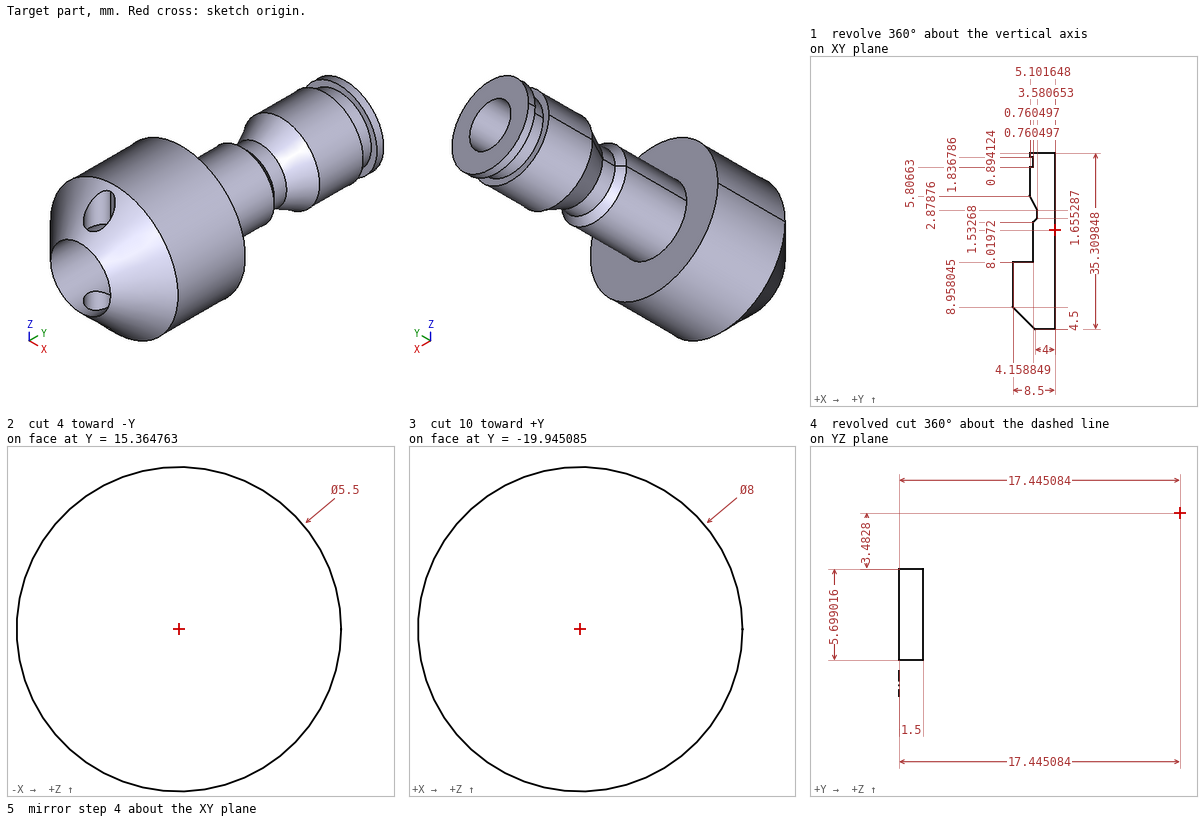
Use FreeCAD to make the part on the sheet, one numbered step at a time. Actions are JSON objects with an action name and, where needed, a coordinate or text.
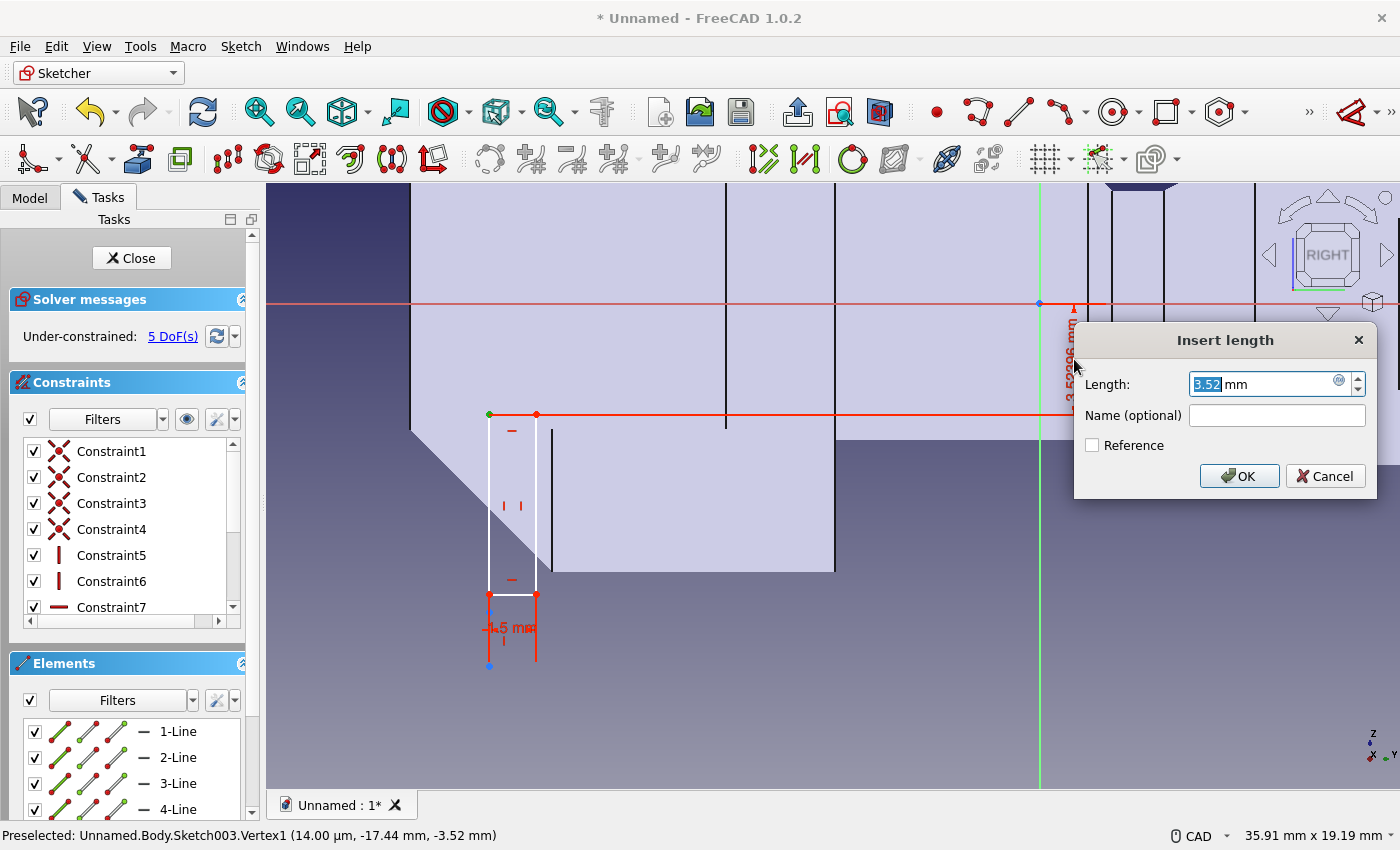
{"action": "type", "text": "3.4828"}
{"action": "key", "text": "Return"}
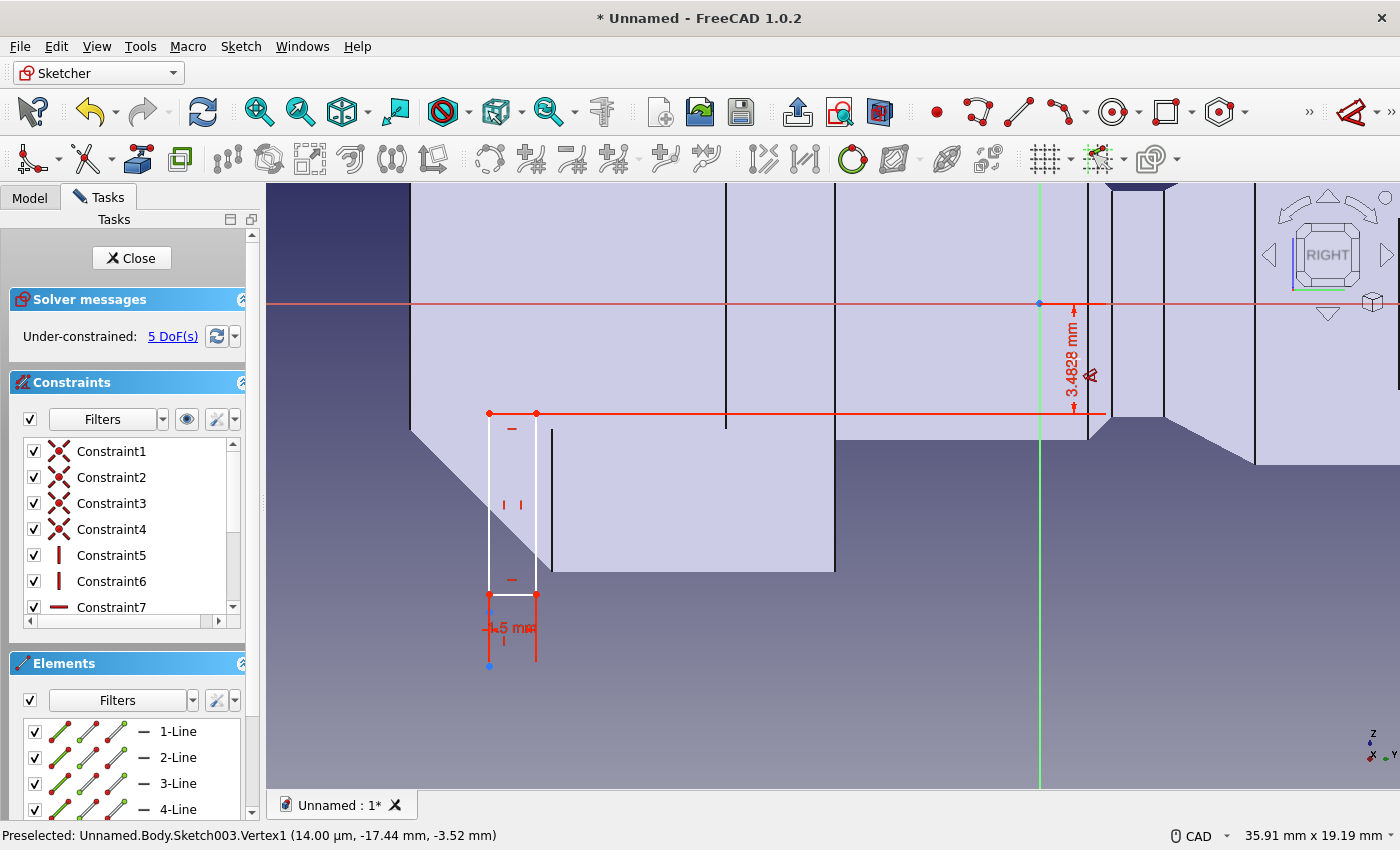
{"action": "left_click", "coordinate": [489, 468]}
{"action": "left_click", "coordinate": [455, 504]}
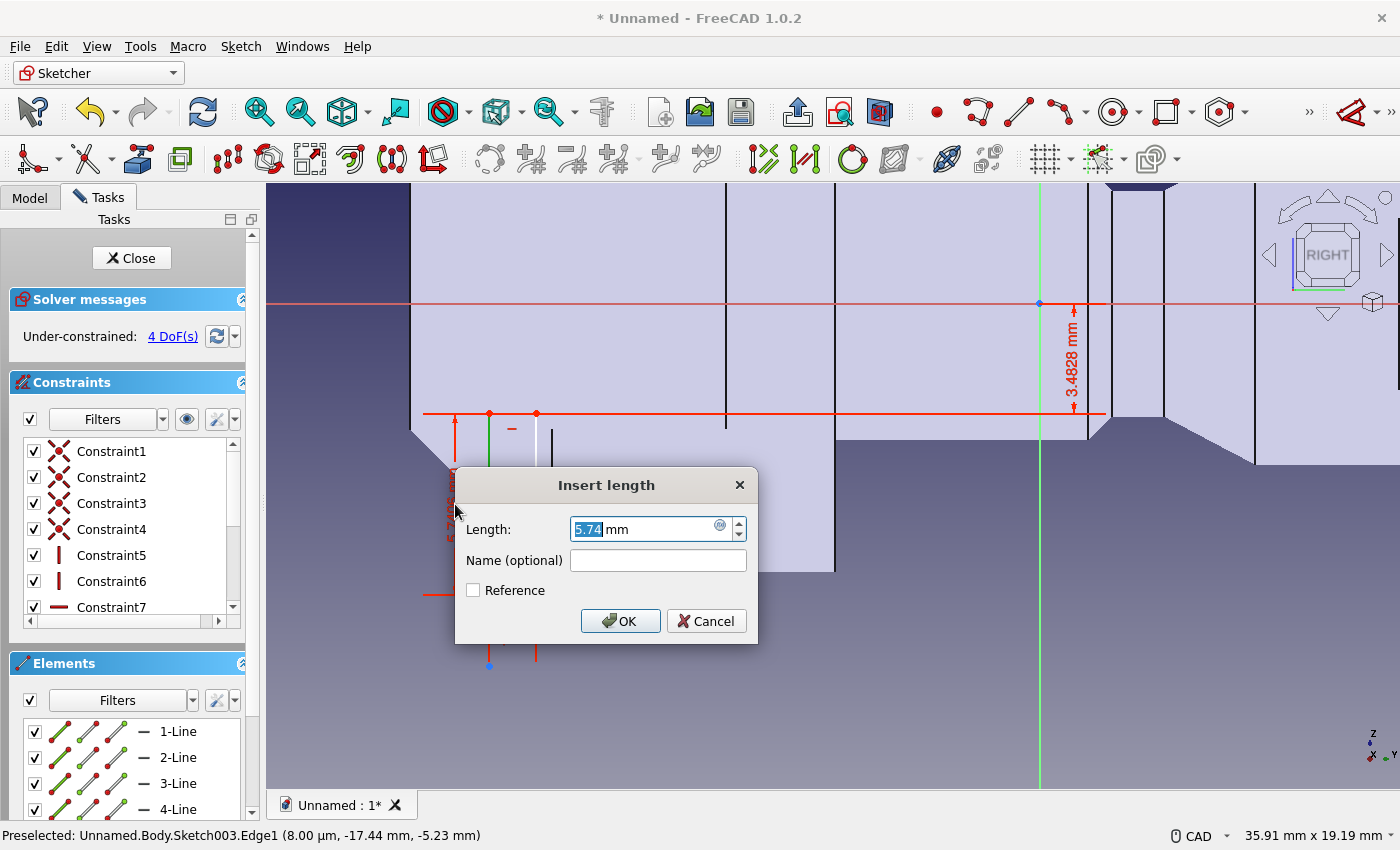
{"action": "type", "text": "5.699016"}
{"action": "key", "text": "Return"}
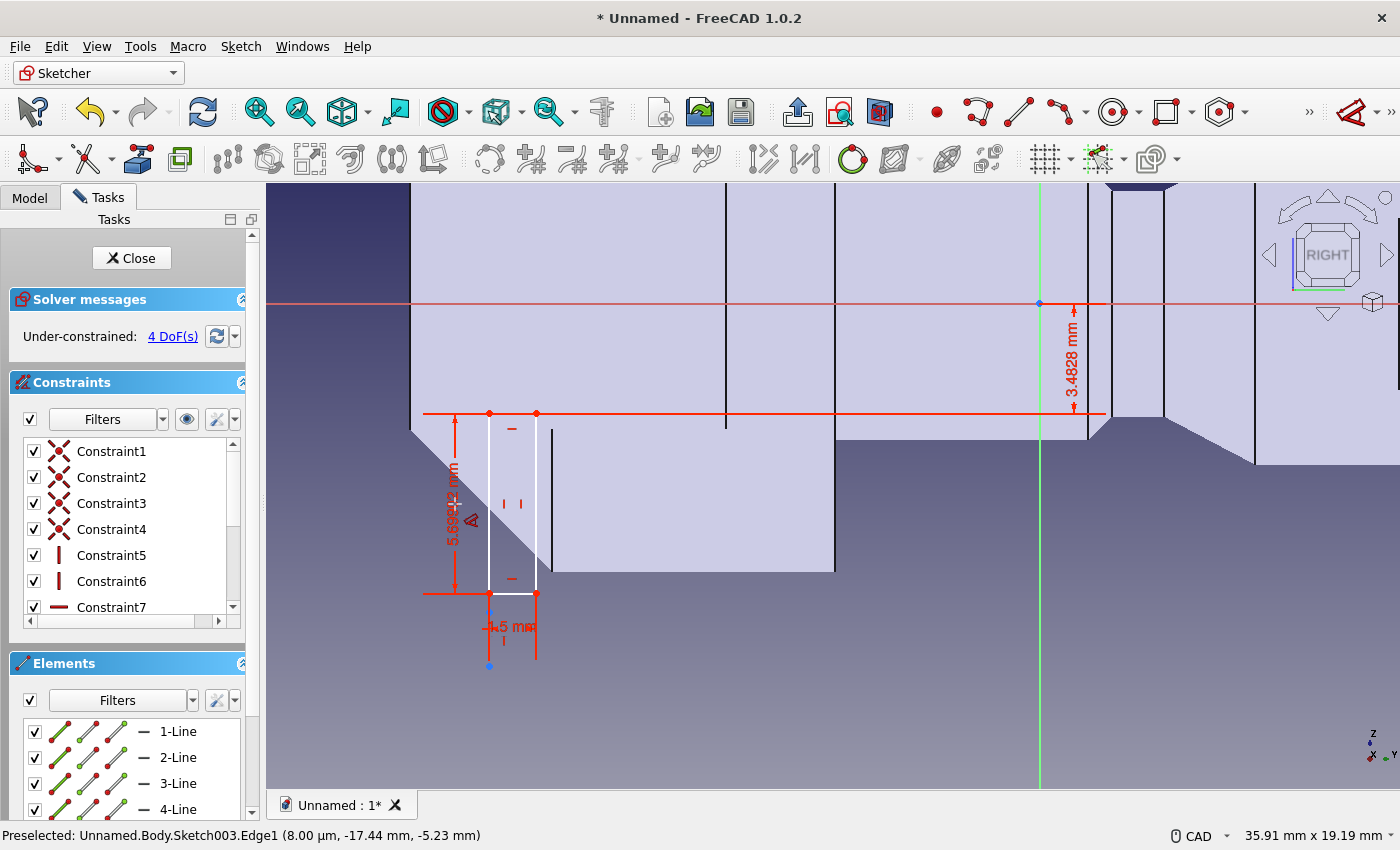
{"action": "left_click", "coordinate": [489, 414]}
{"action": "left_click", "coordinate": [764, 270]}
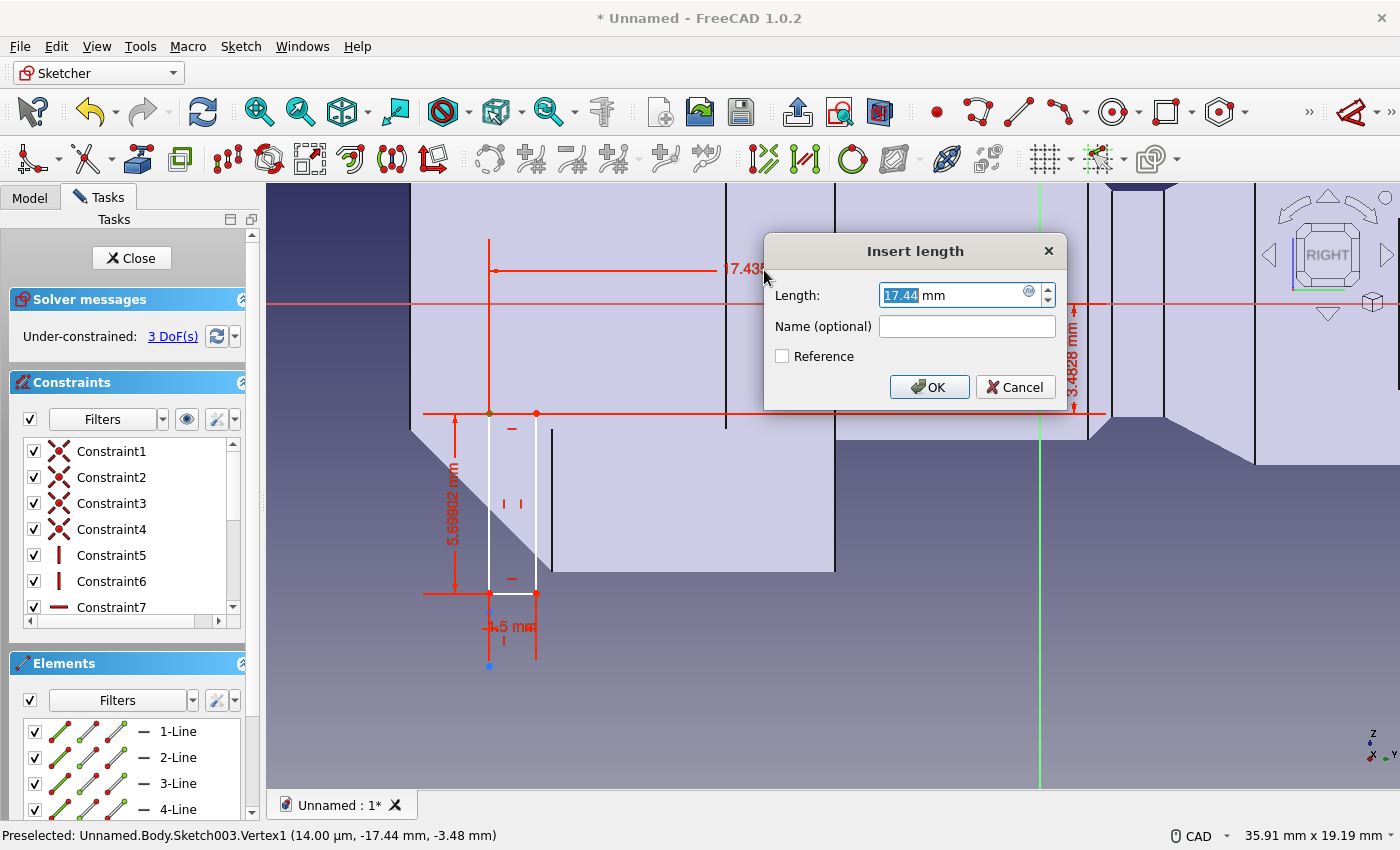
{"action": "type", "text": "17.445084"}
{"action": "key", "text": "Return"}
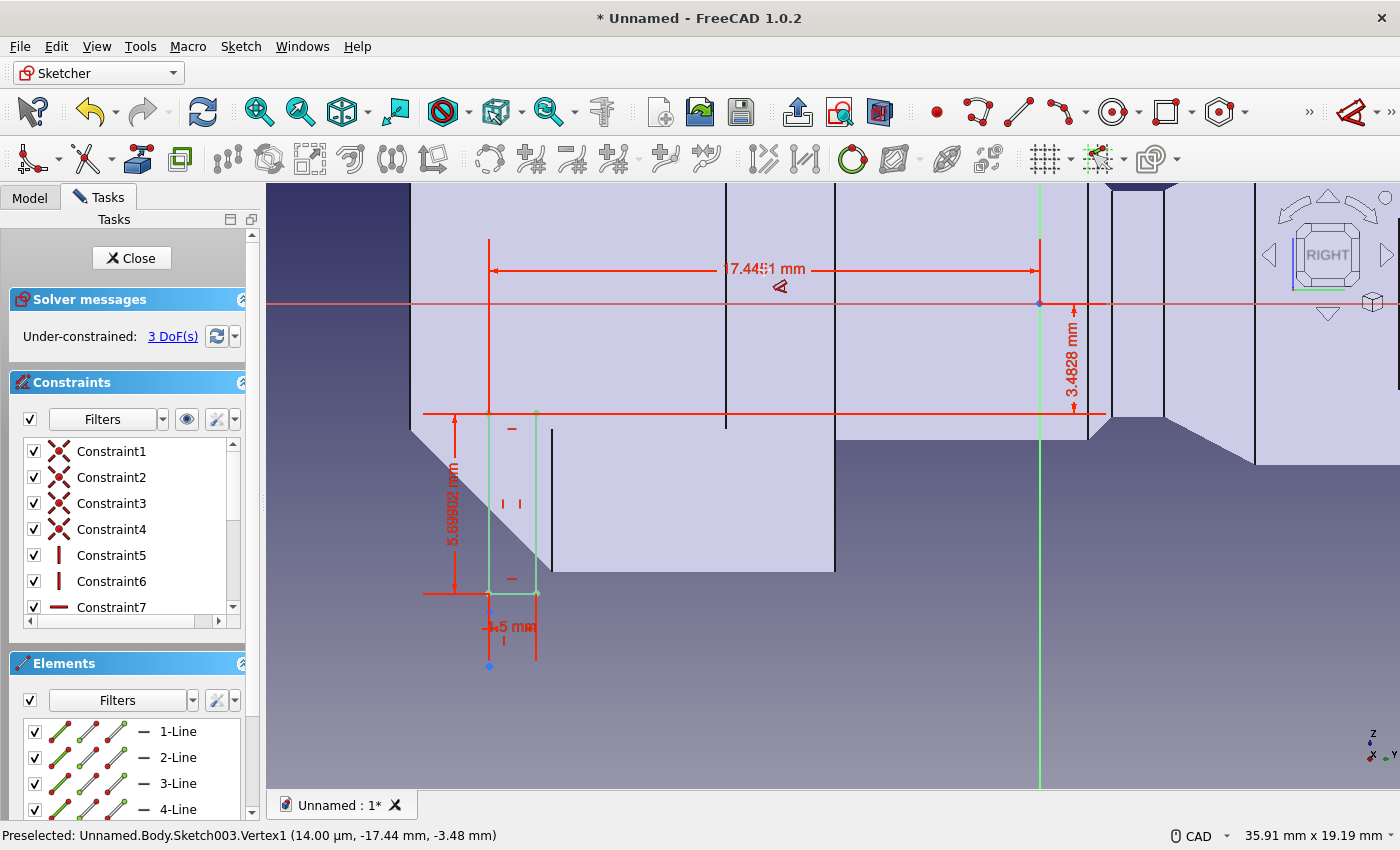
{"action": "left_click", "coordinate": [489, 613]}
{"action": "left_click", "coordinate": [638, 270]}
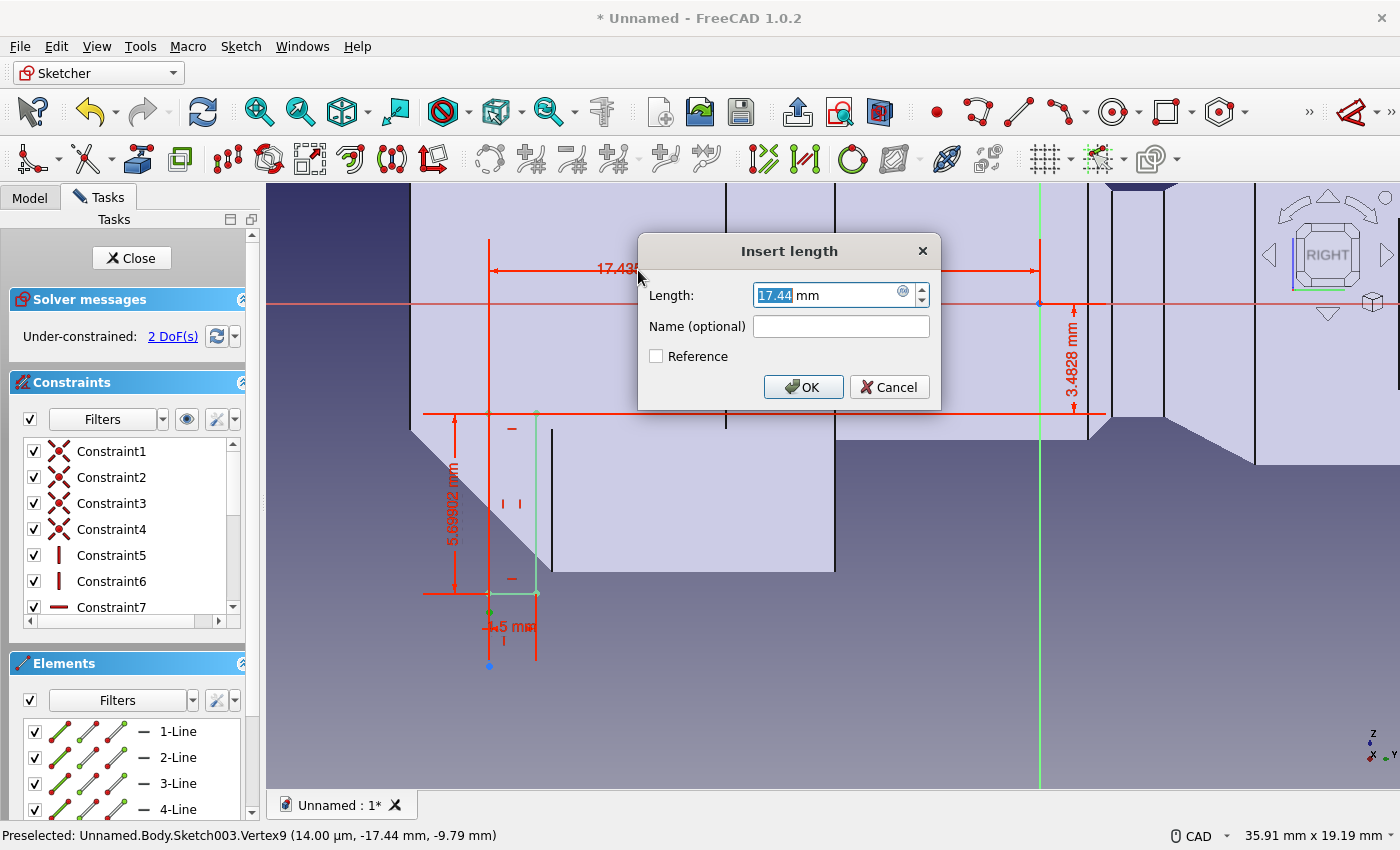
{"action": "type", "text": "17.445084"}
{"action": "key", "text": "Return"}
{"action": "key", "text": "Escape"}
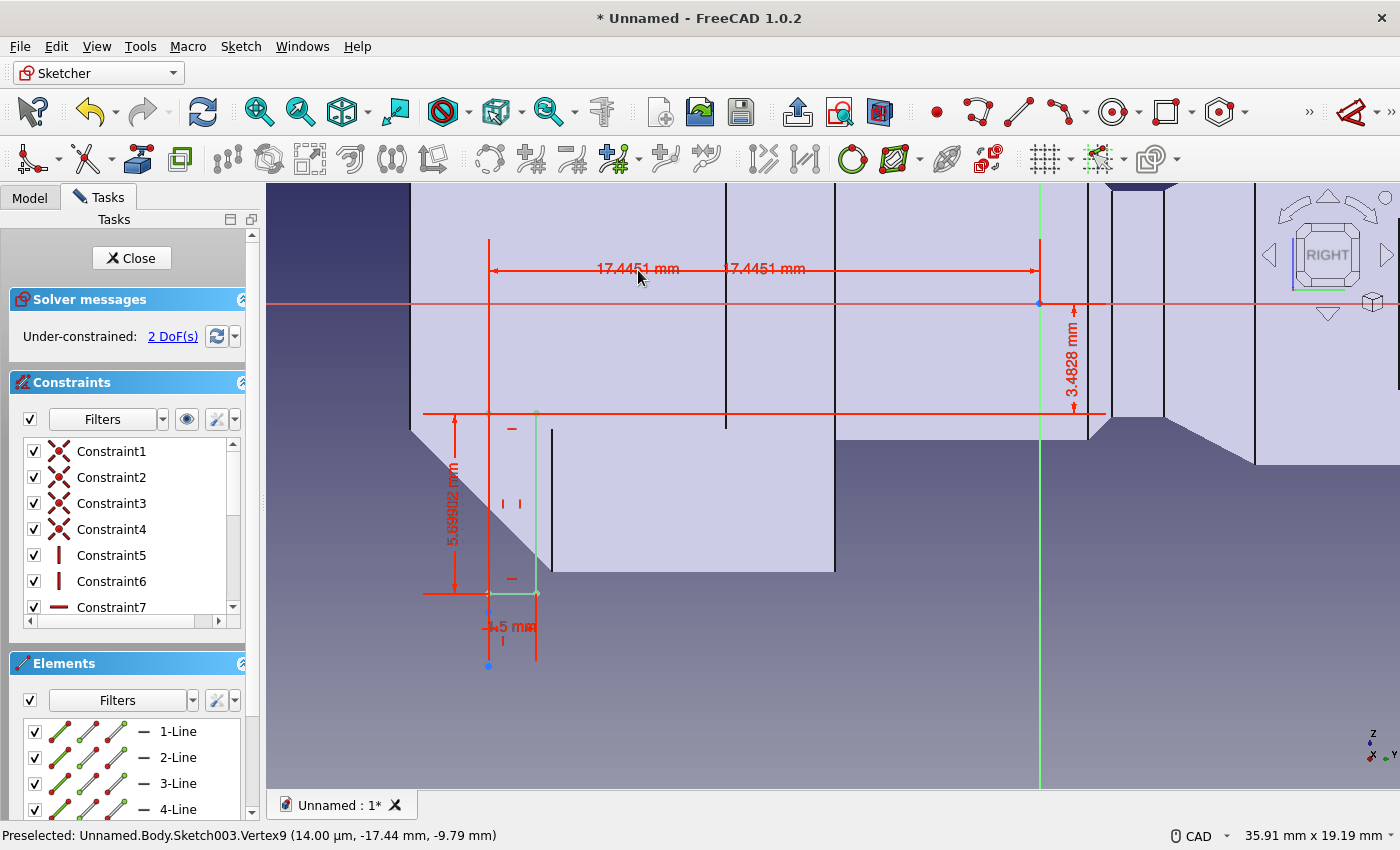
{"action": "left_click", "coordinate": [132, 258]}